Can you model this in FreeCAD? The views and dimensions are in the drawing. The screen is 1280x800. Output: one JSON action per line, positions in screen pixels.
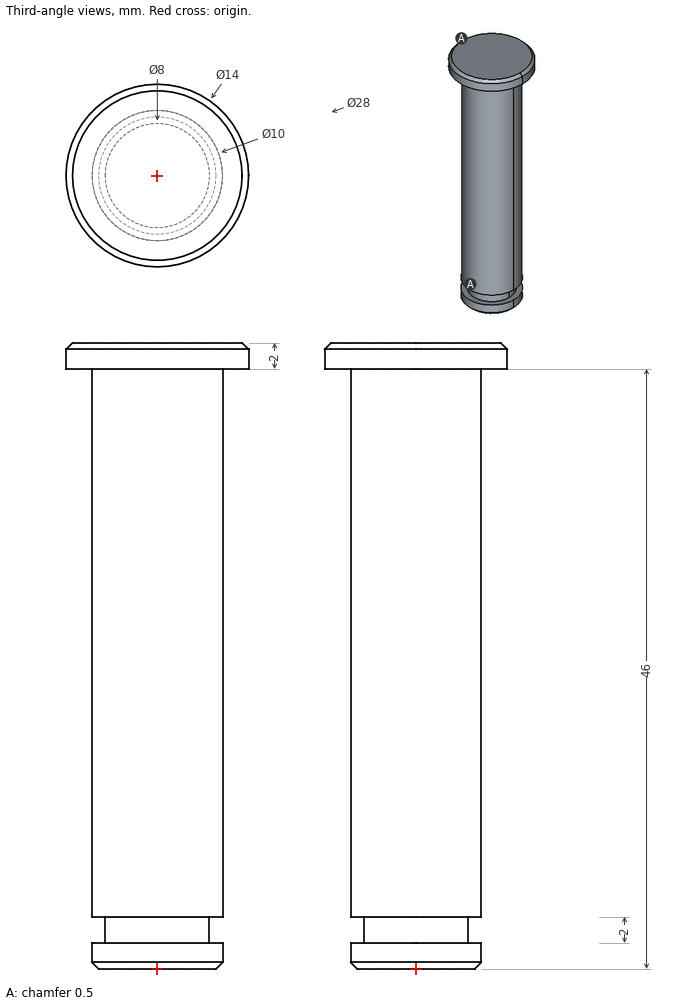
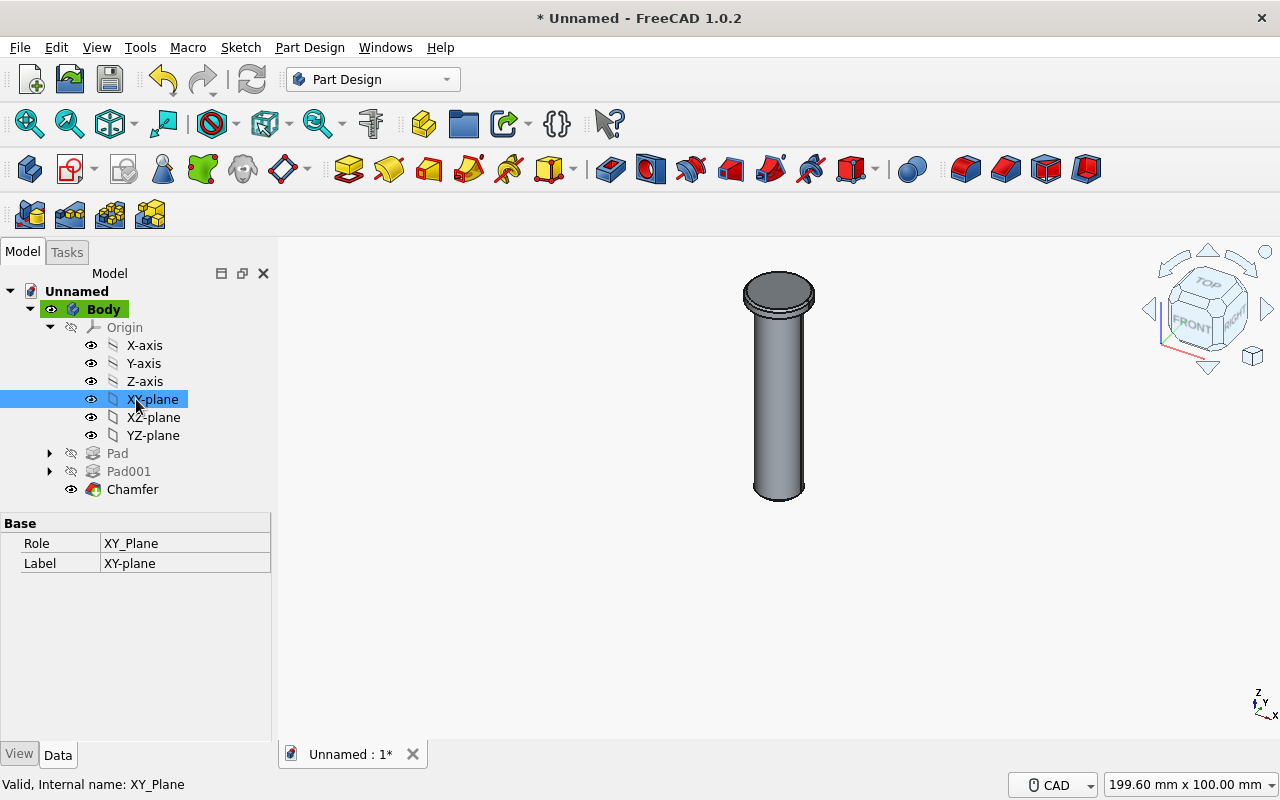
{"action": "left_click", "coordinate": [284, 170]}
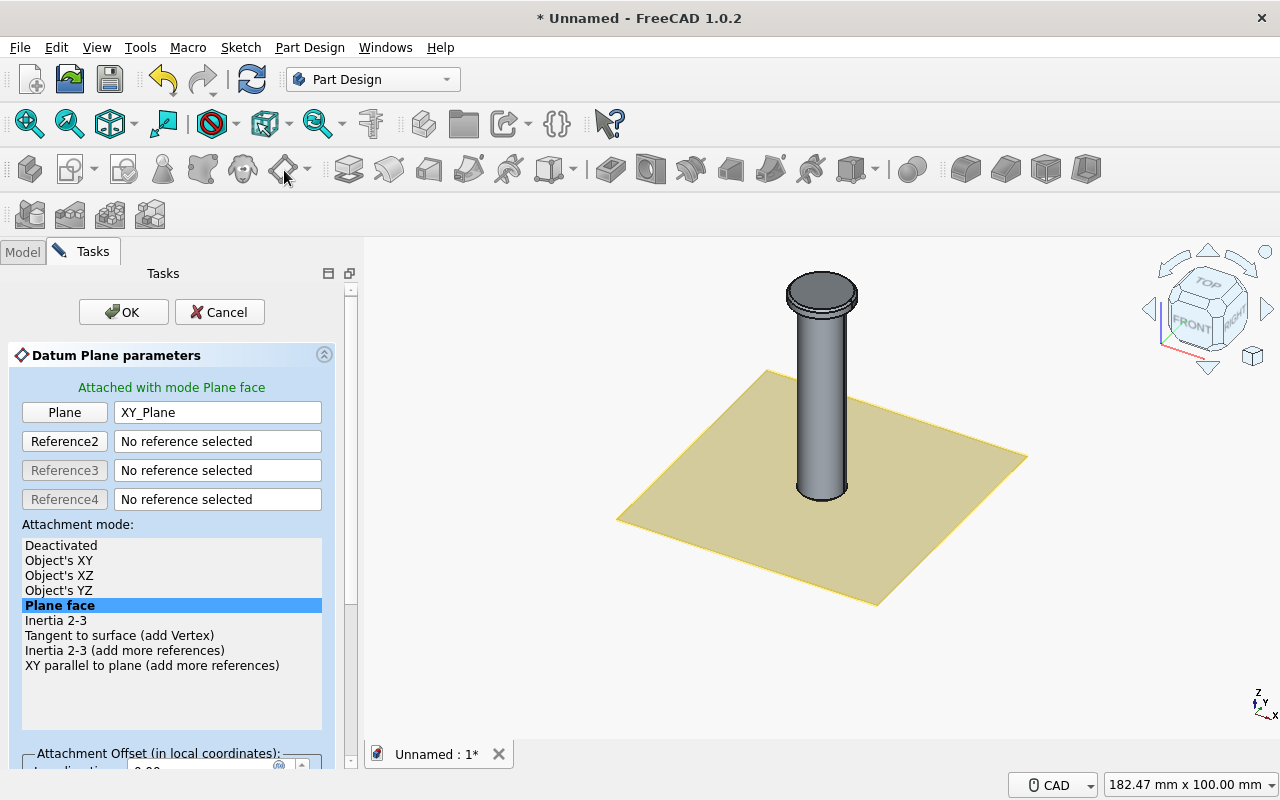
{"action": "scroll", "coordinate": [351, 526], "scroll_direction": "down", "scroll_amount": 3}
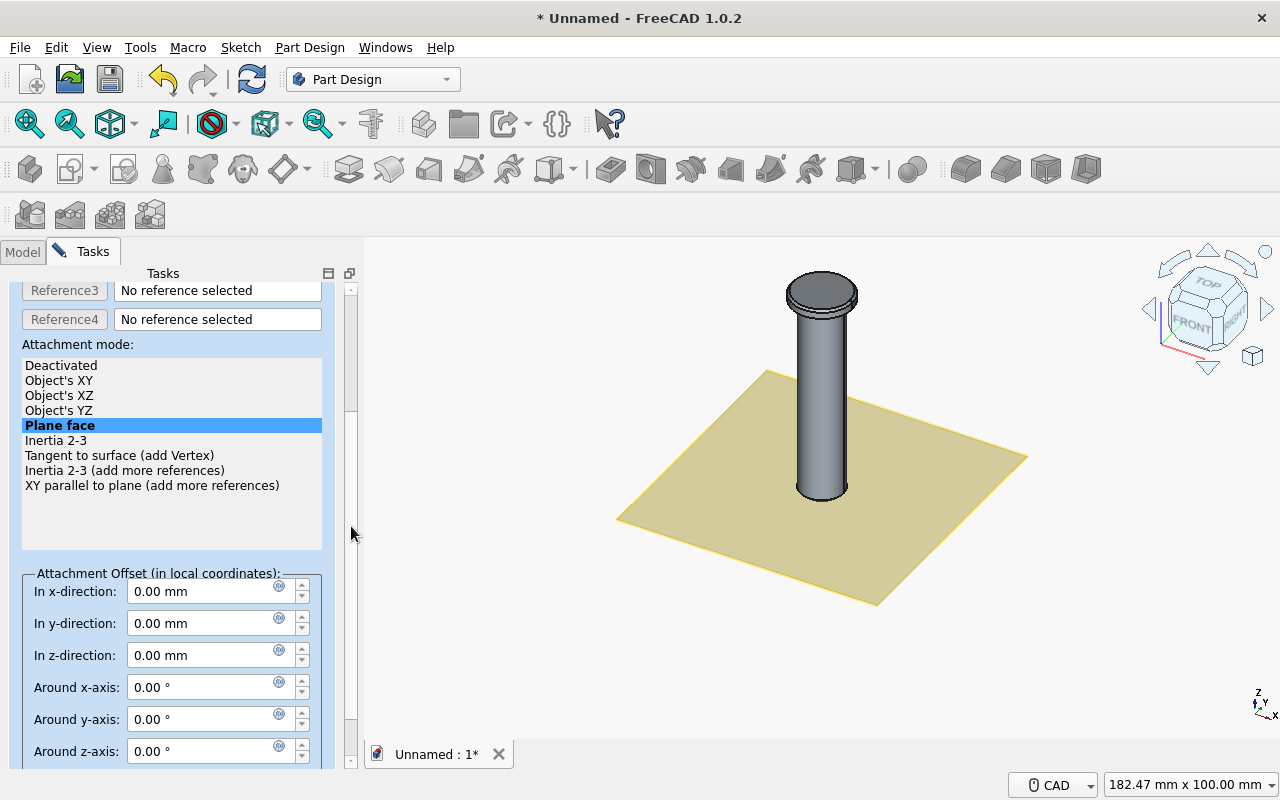
{"action": "triple_click", "coordinate": [210, 655]}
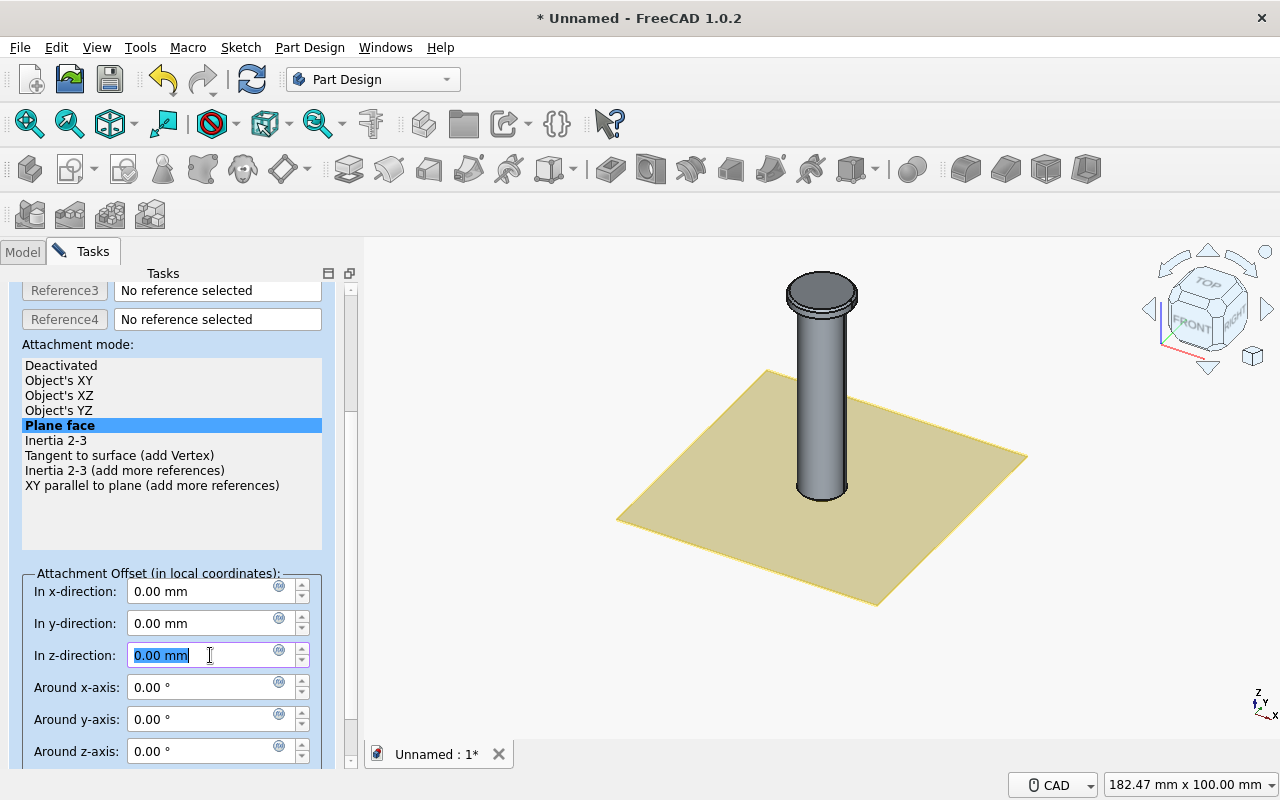
{"action": "type", "text": "2"}
{"action": "key", "text": "Tab"}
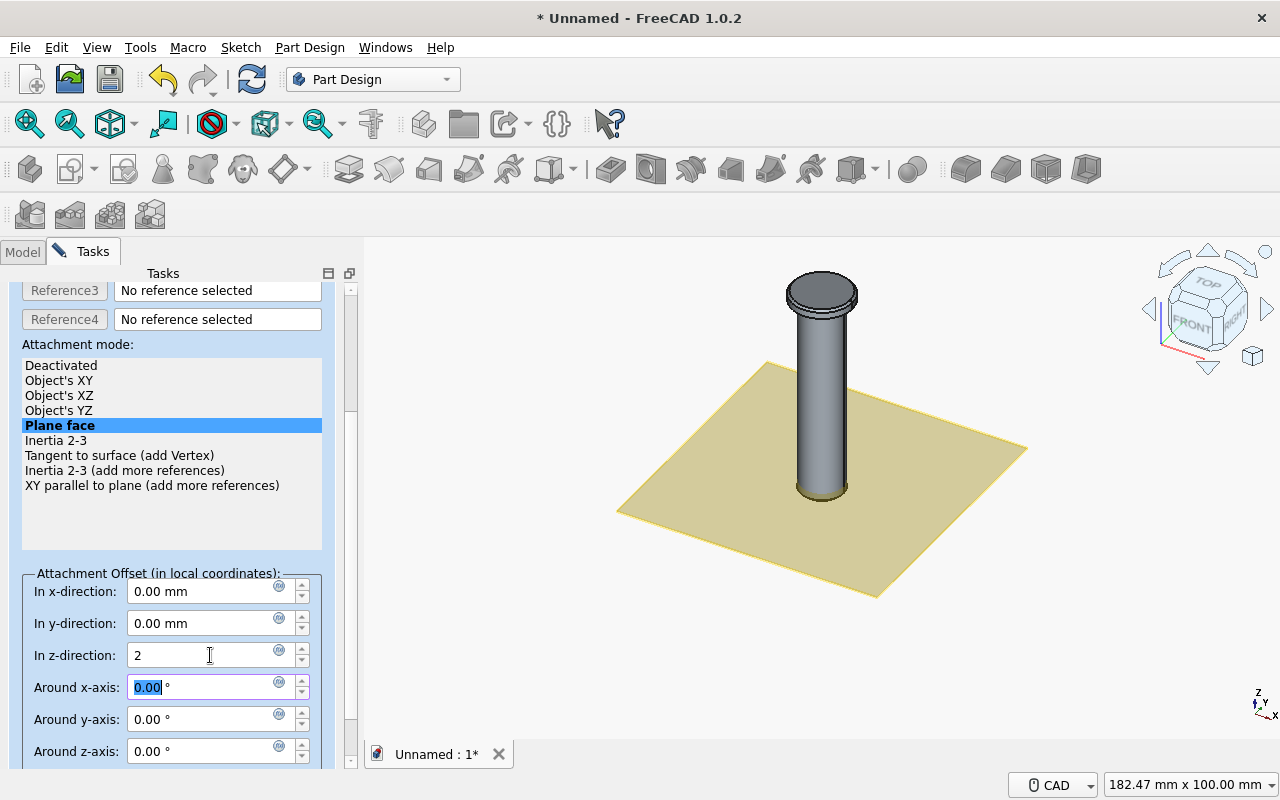
{"action": "scroll", "coordinate": [351, 526], "scroll_direction": "up", "scroll_amount": 4}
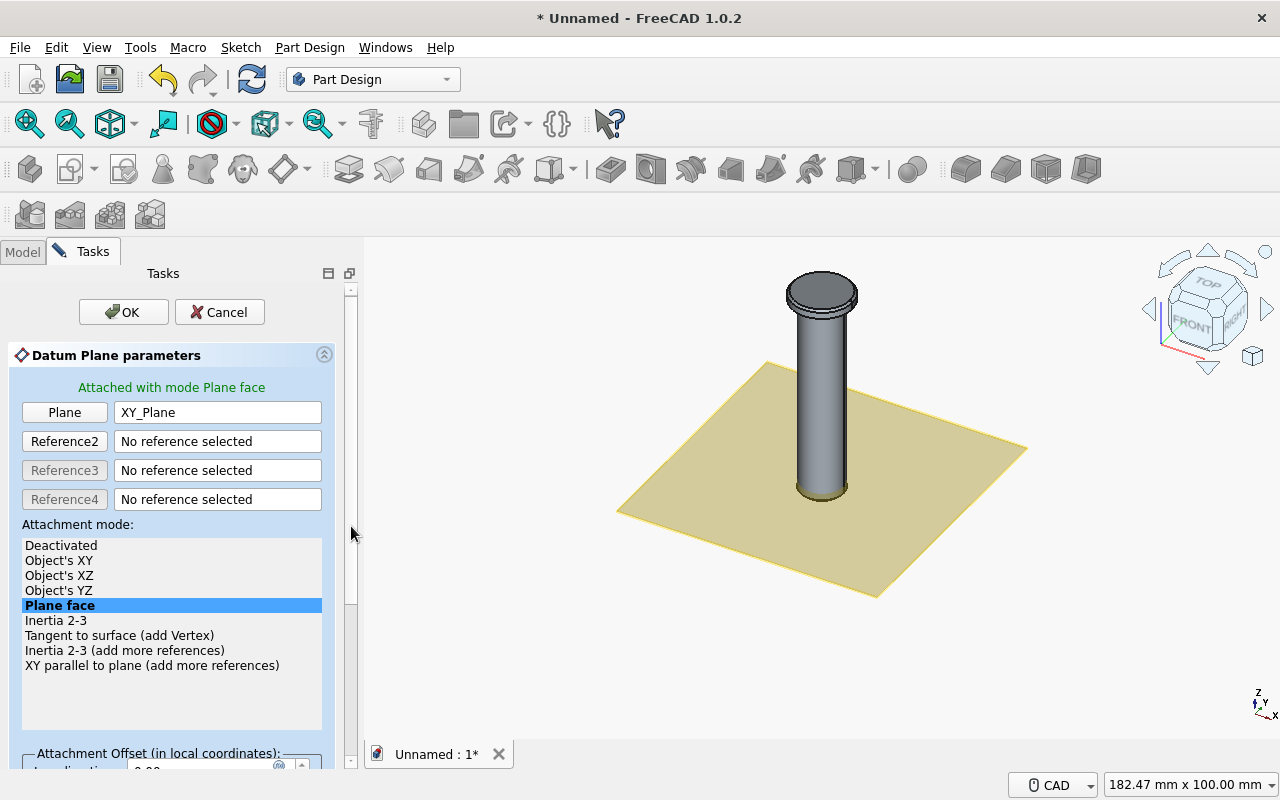
{"action": "left_click", "coordinate": [124, 312]}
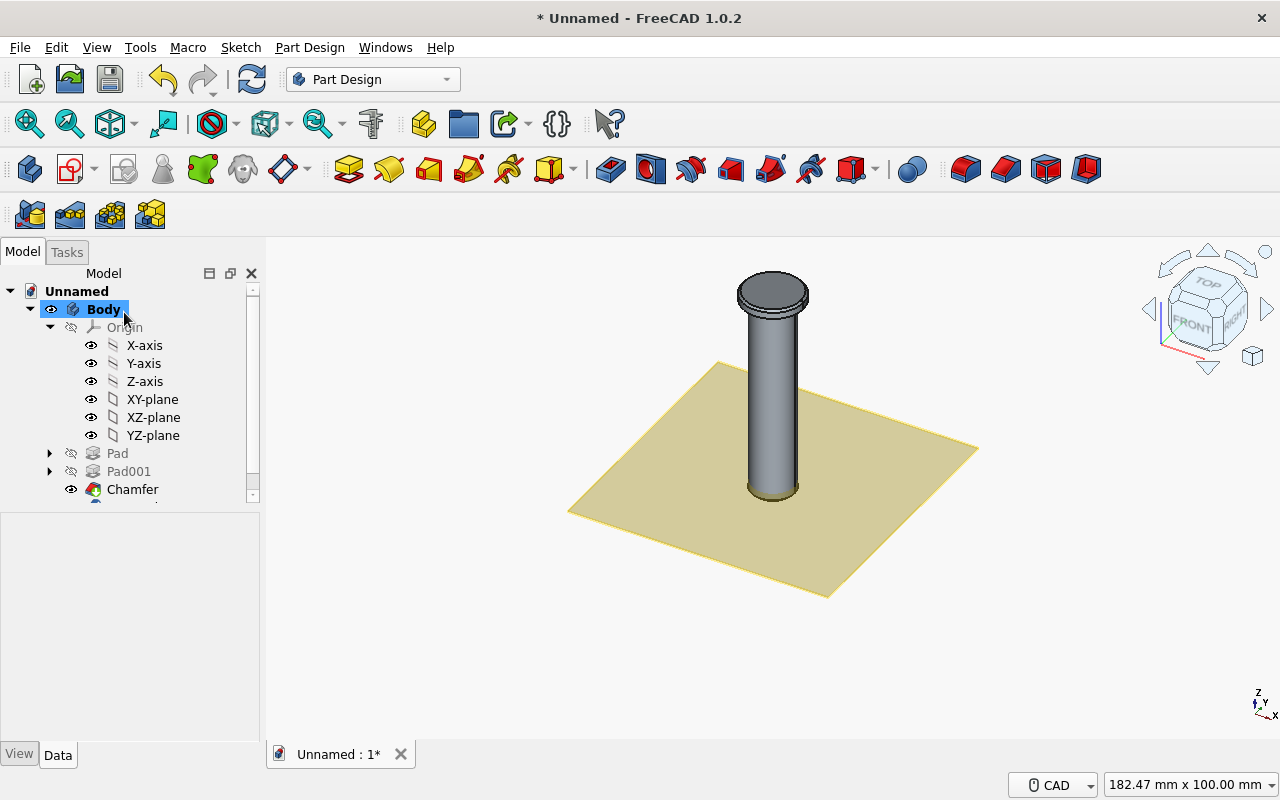
{"action": "scroll", "coordinate": [100, 395], "scroll_direction": "down", "scroll_amount": 3}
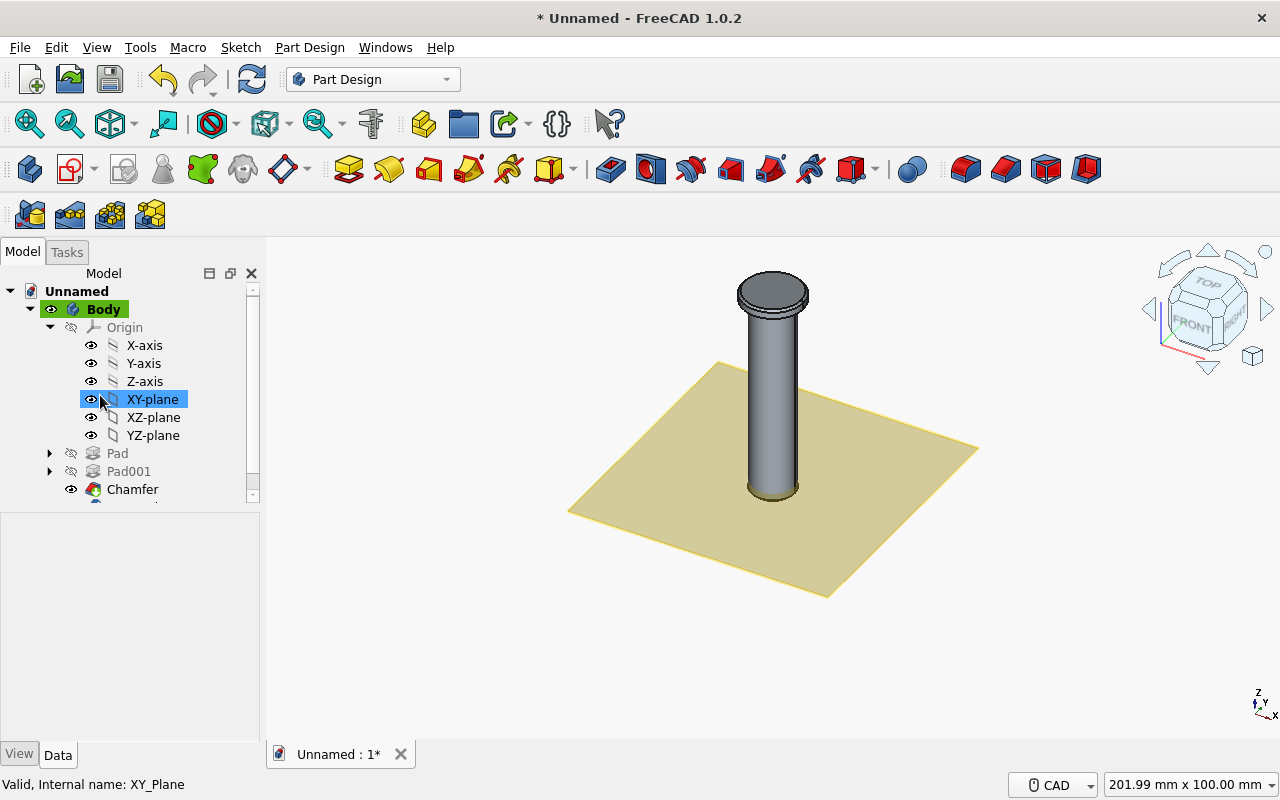
{"action": "left_click", "coordinate": [116, 489]}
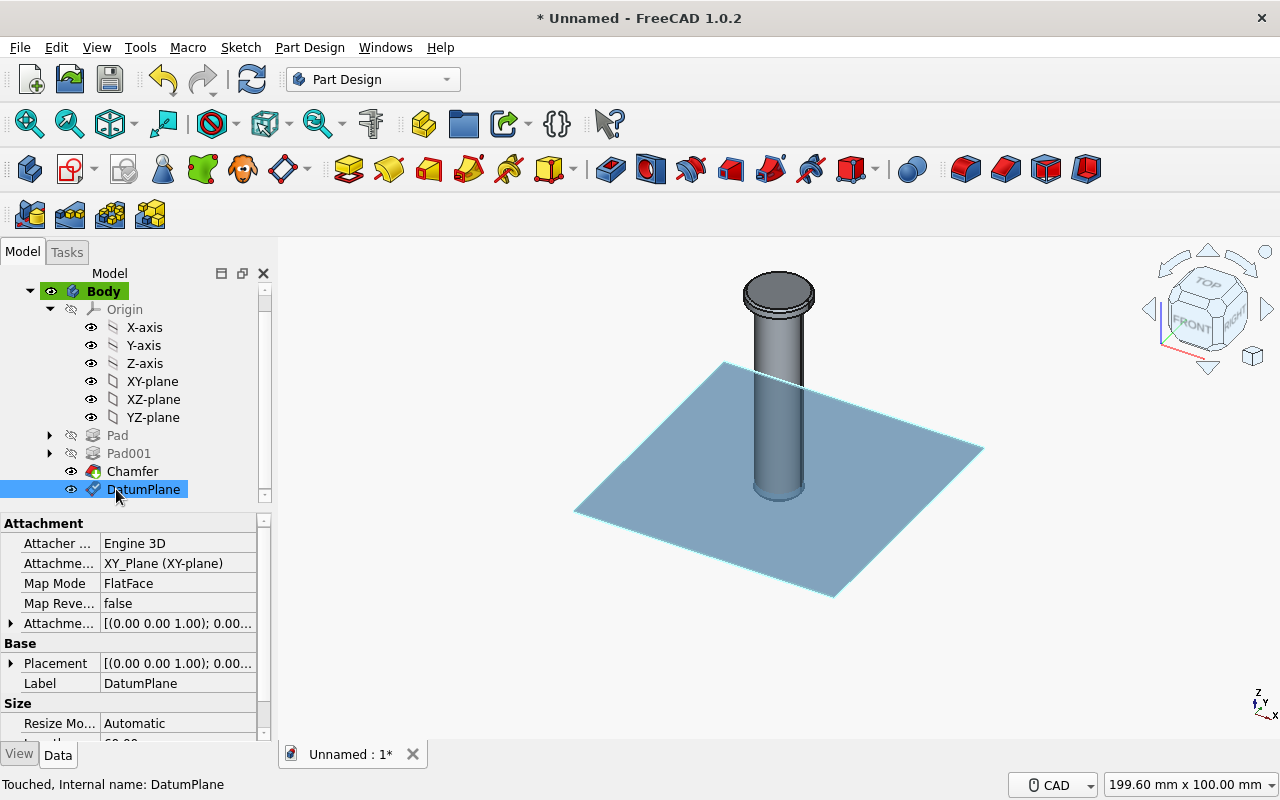
{"action": "left_click", "coordinate": [70, 170]}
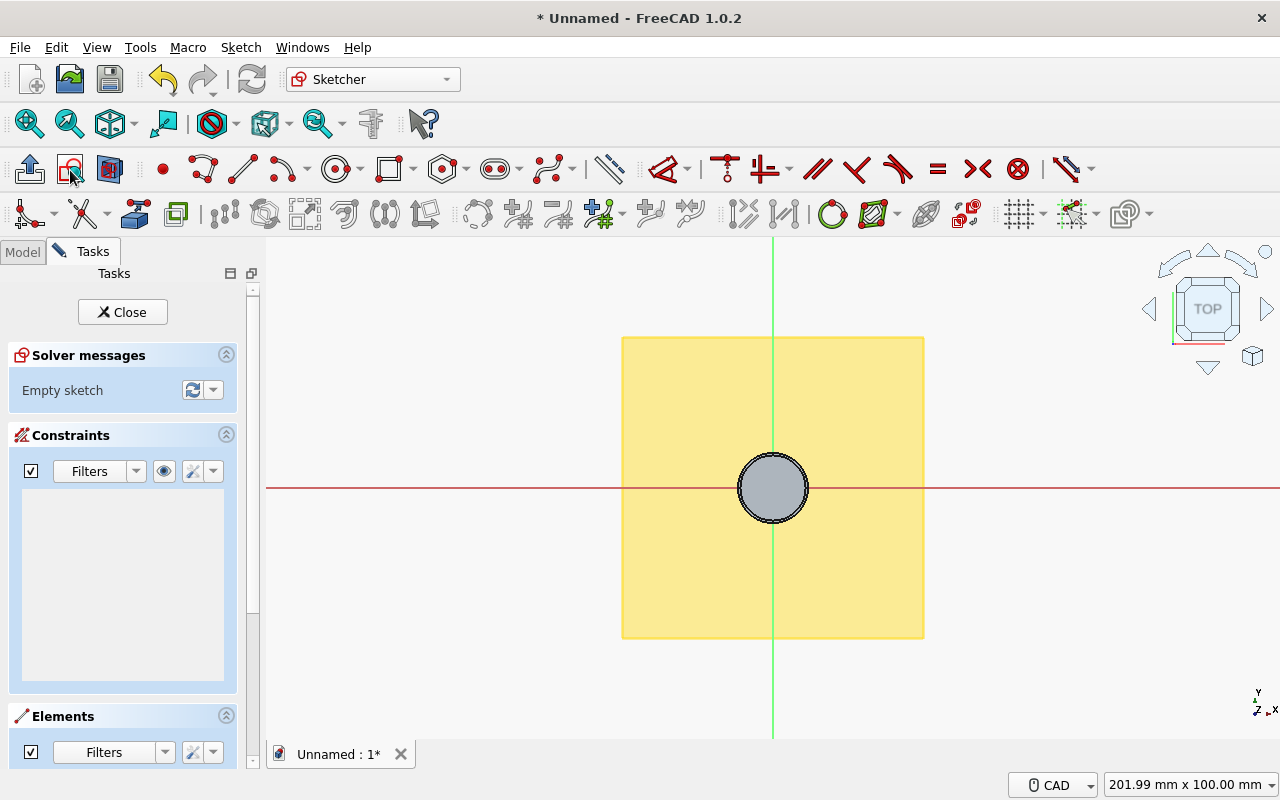
{"action": "key", "text": "q s"}